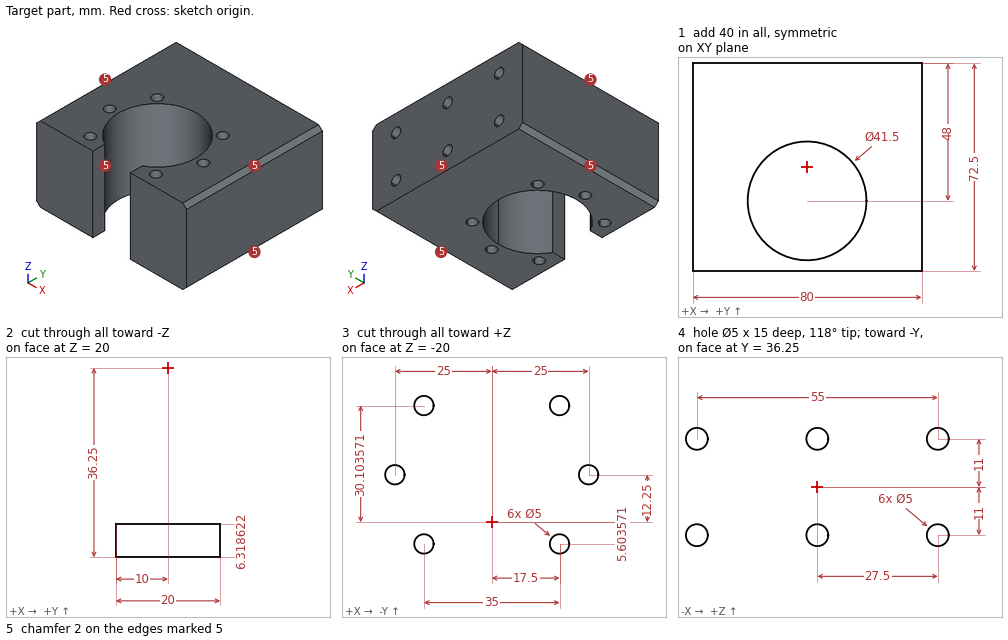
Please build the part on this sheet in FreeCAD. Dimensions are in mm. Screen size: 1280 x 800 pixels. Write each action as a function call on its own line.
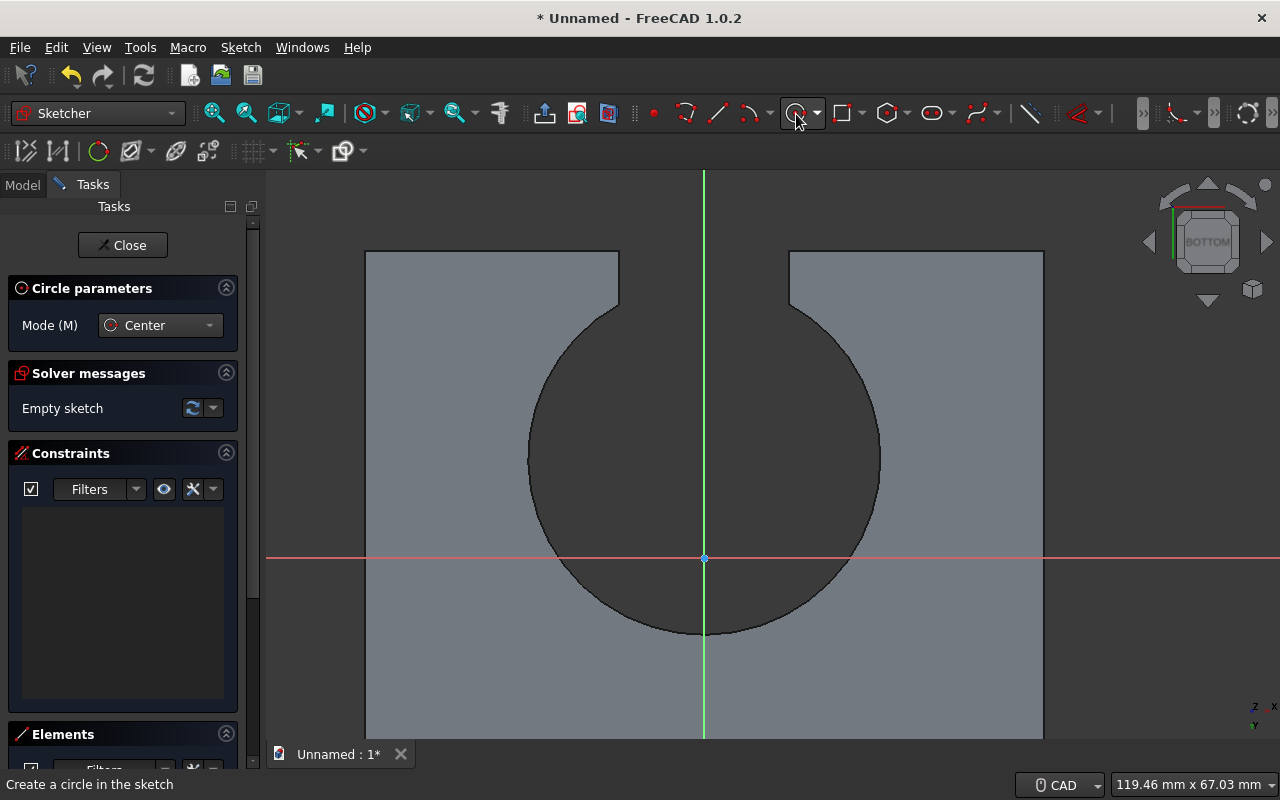
click(853, 606)
move(868, 591)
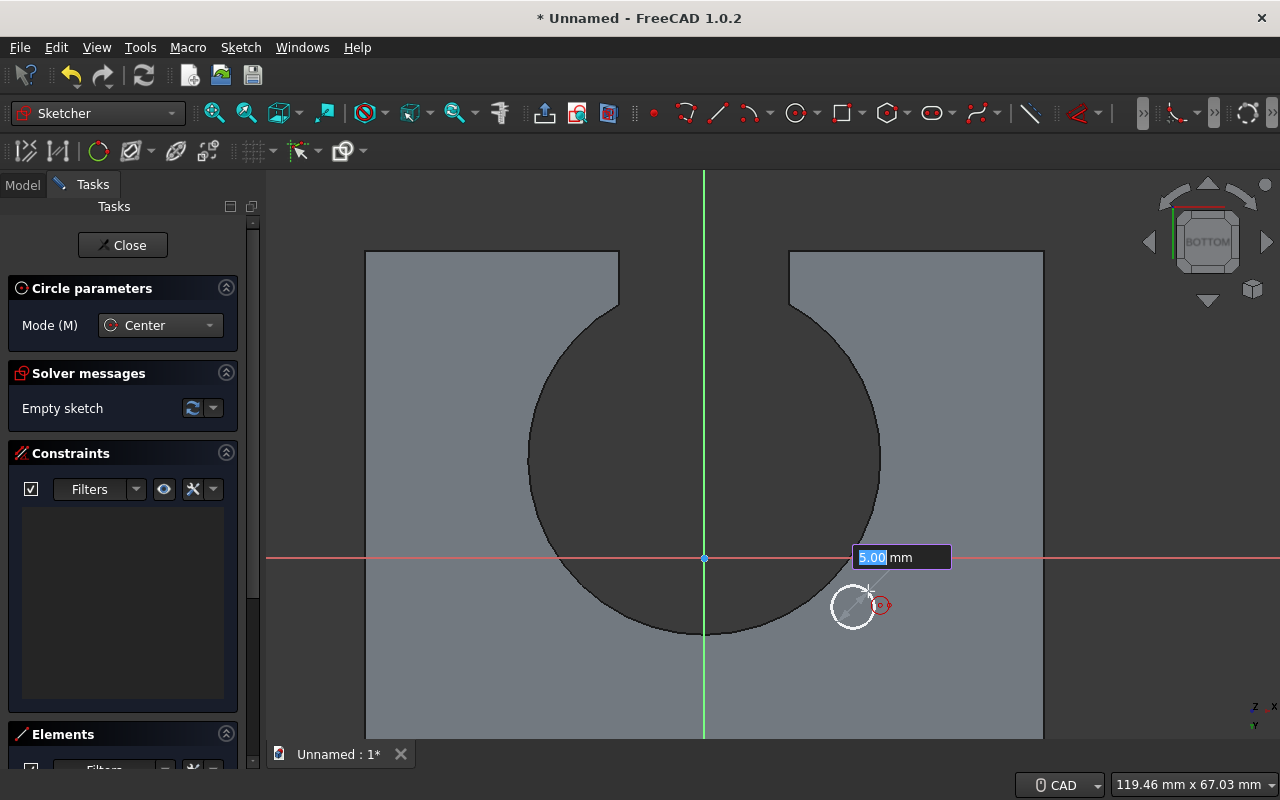
text(5)
key(Return)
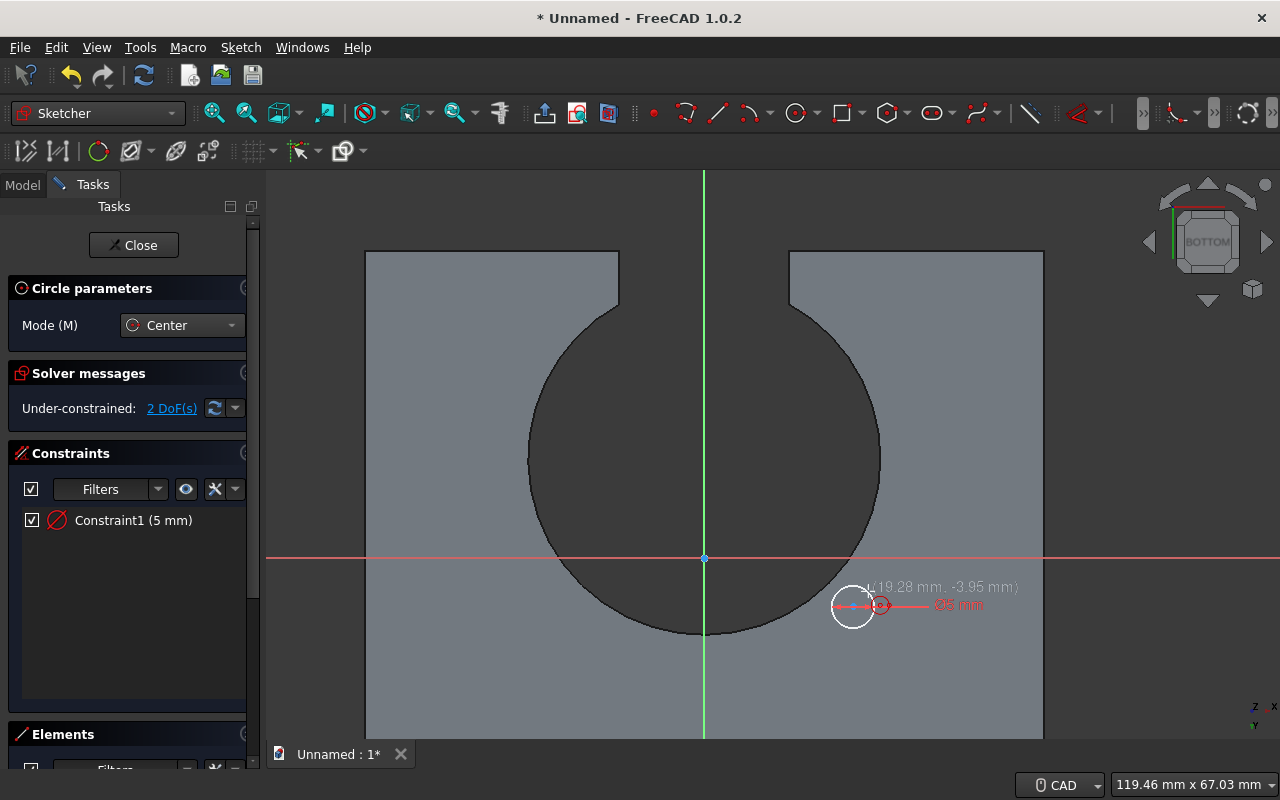
click(556, 606)
move(571, 591)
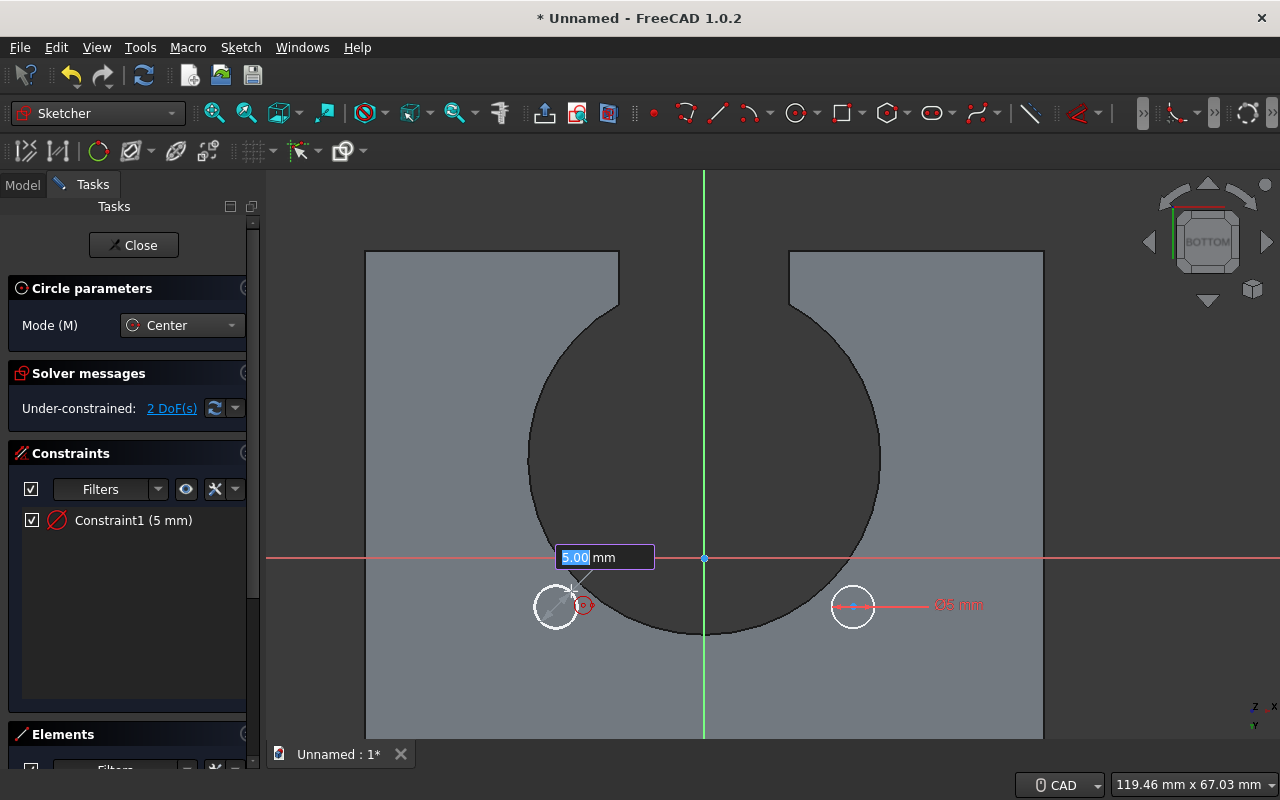
text(5)
key(Return)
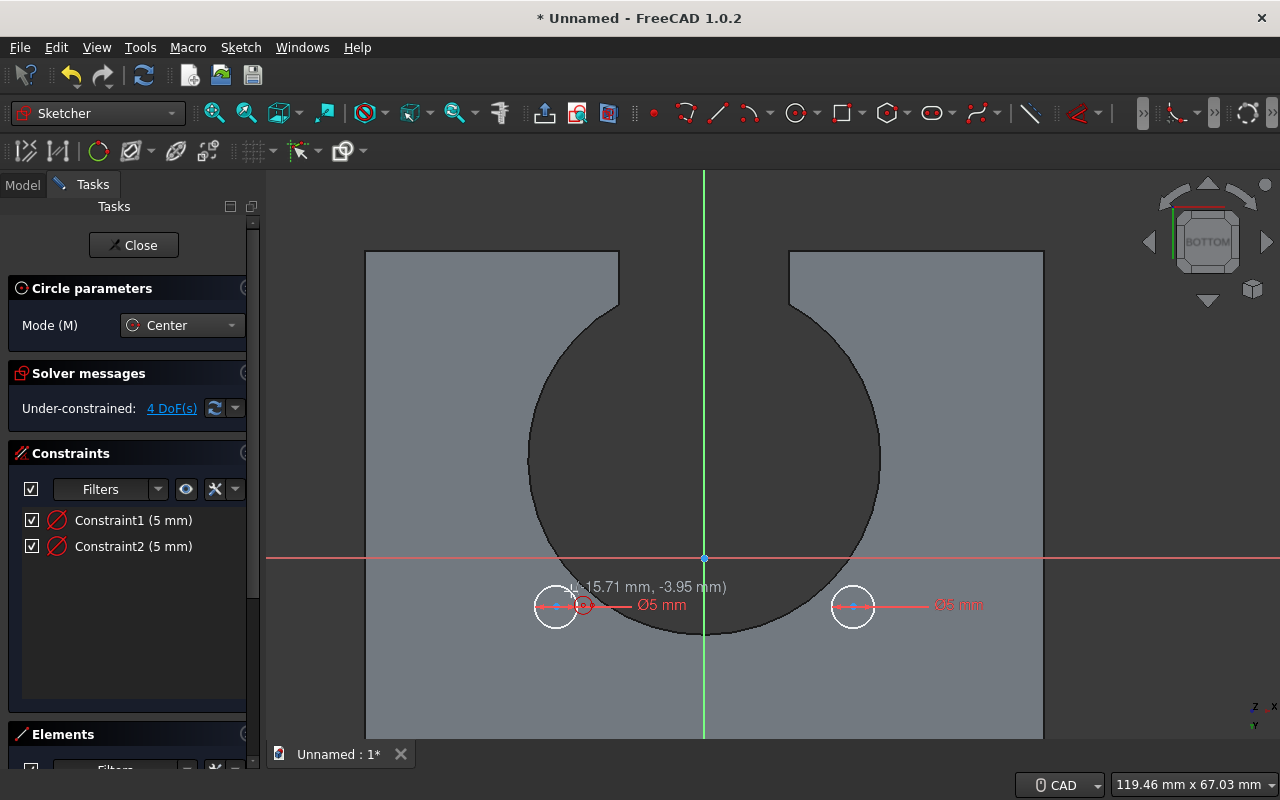
click(556, 303)
move(571, 288)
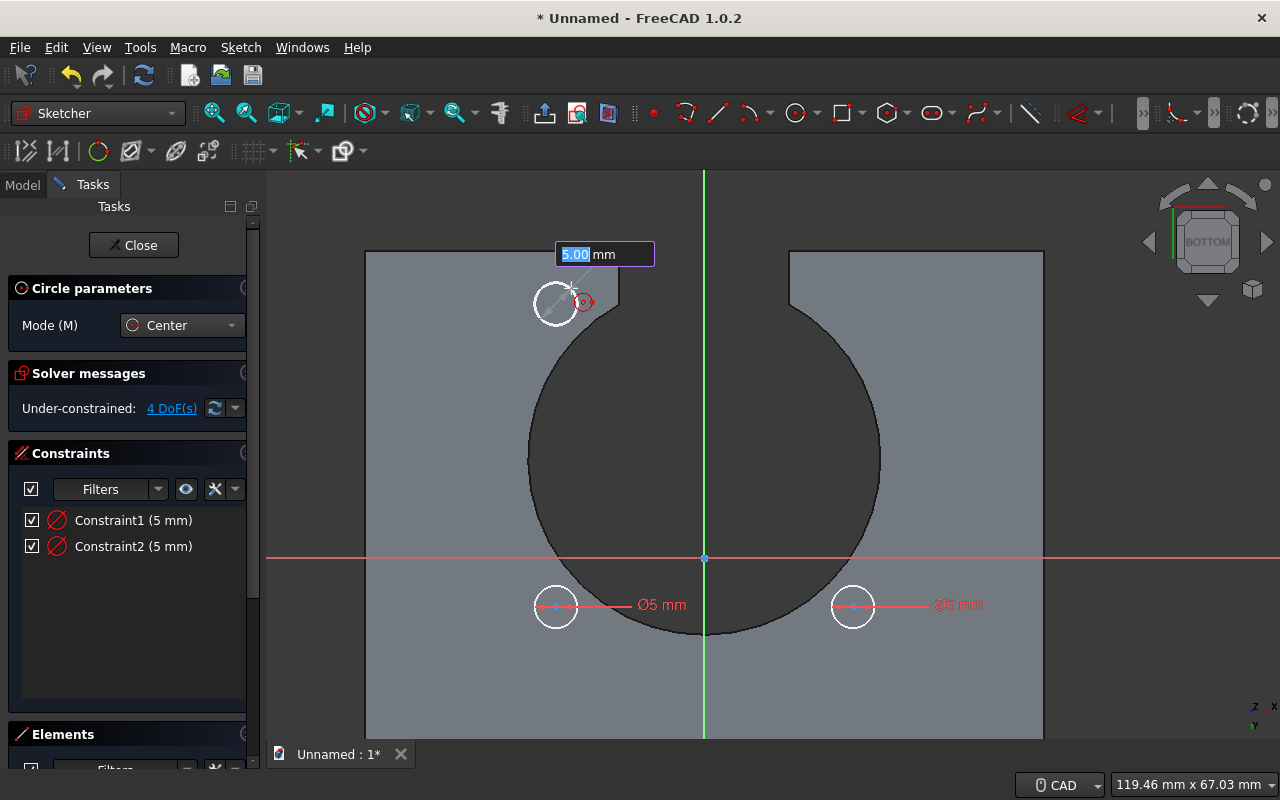
text(5)
key(Return)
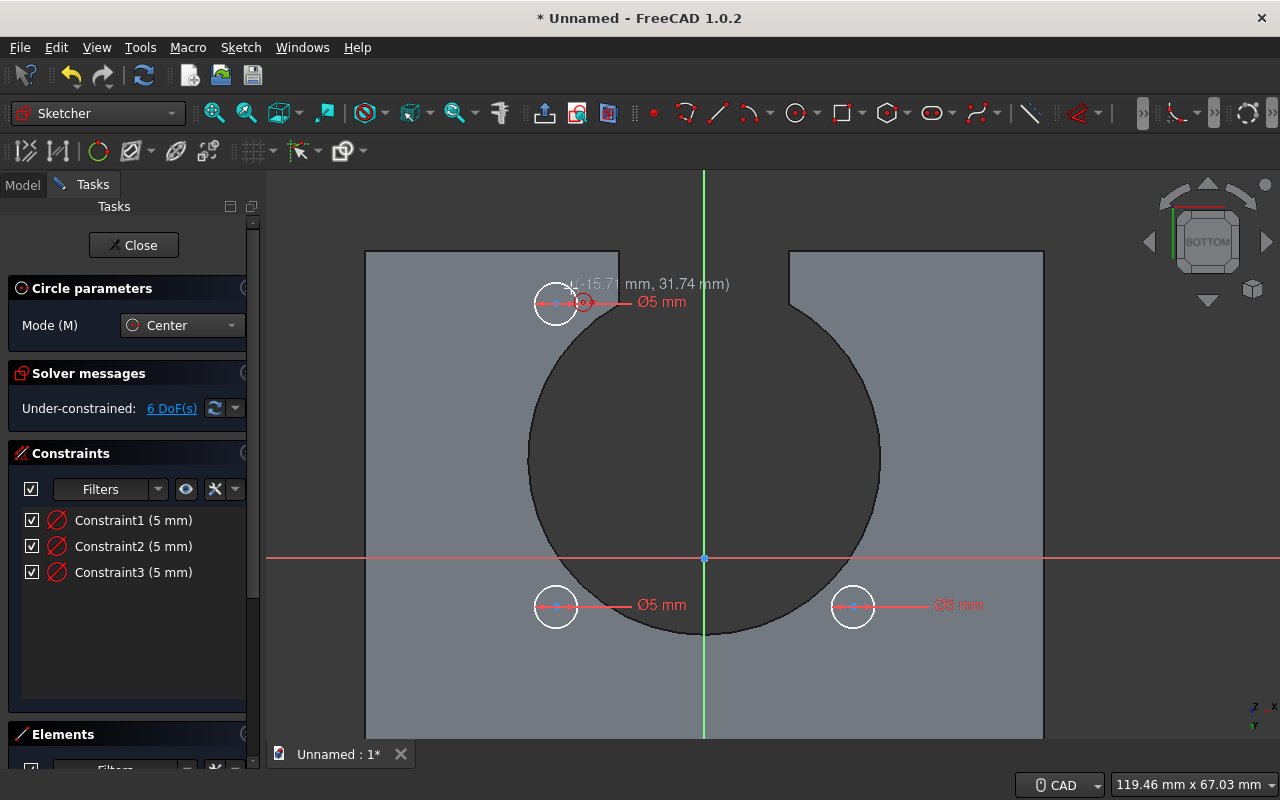
click(853, 303)
move(868, 288)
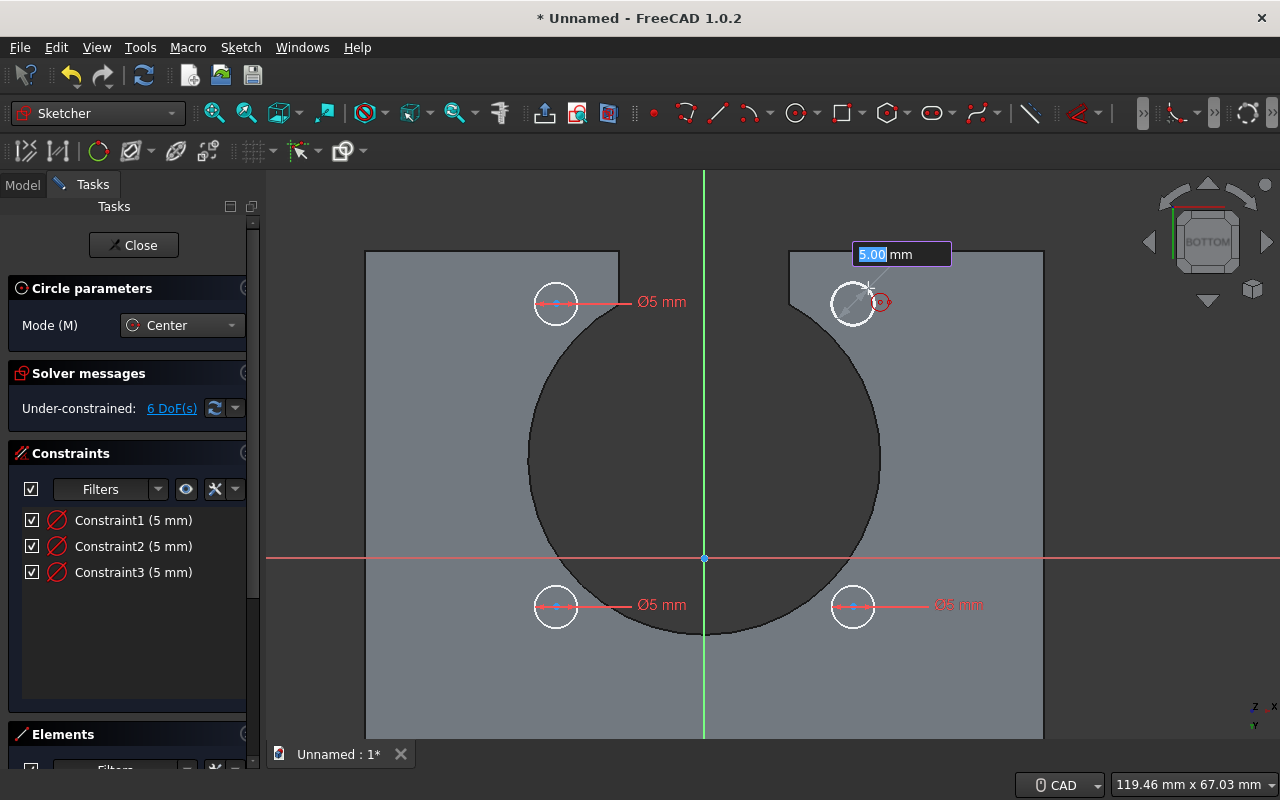
text(5)
key(Return)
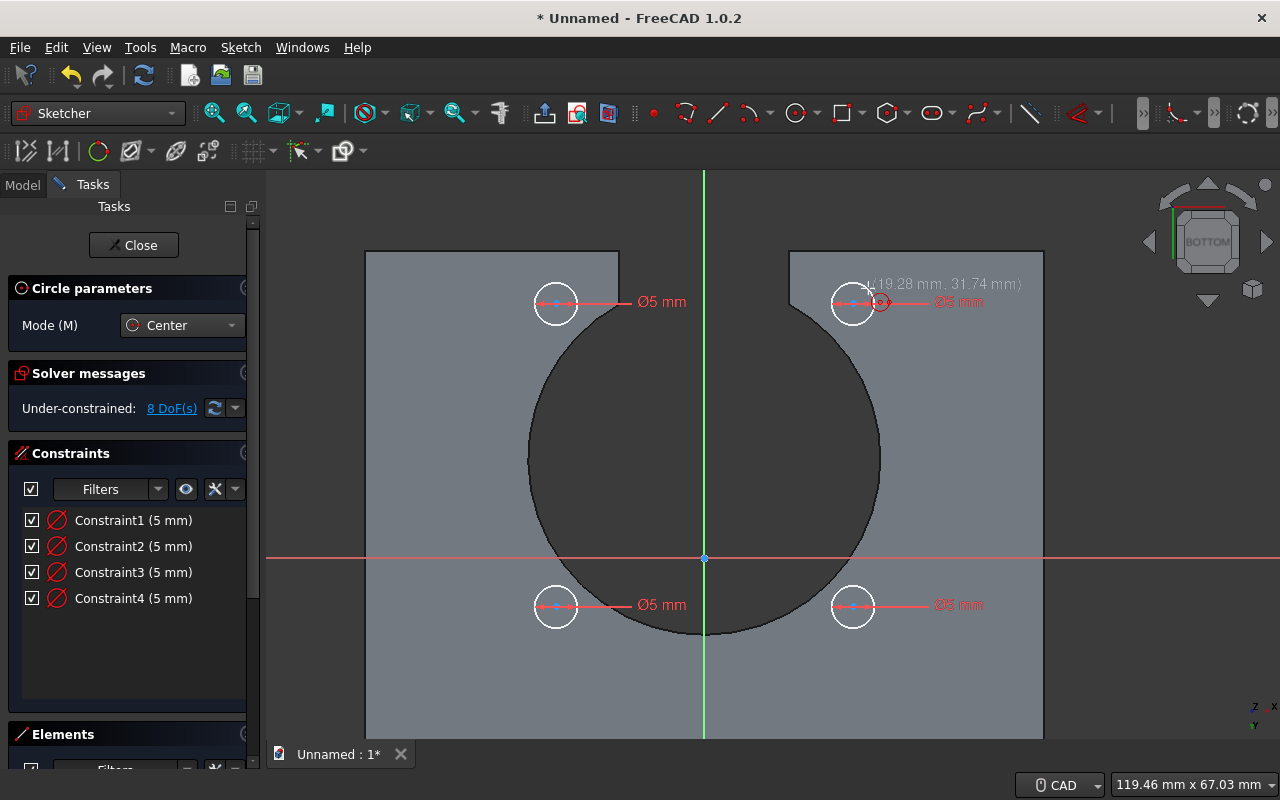
click(917, 454)
move(932, 439)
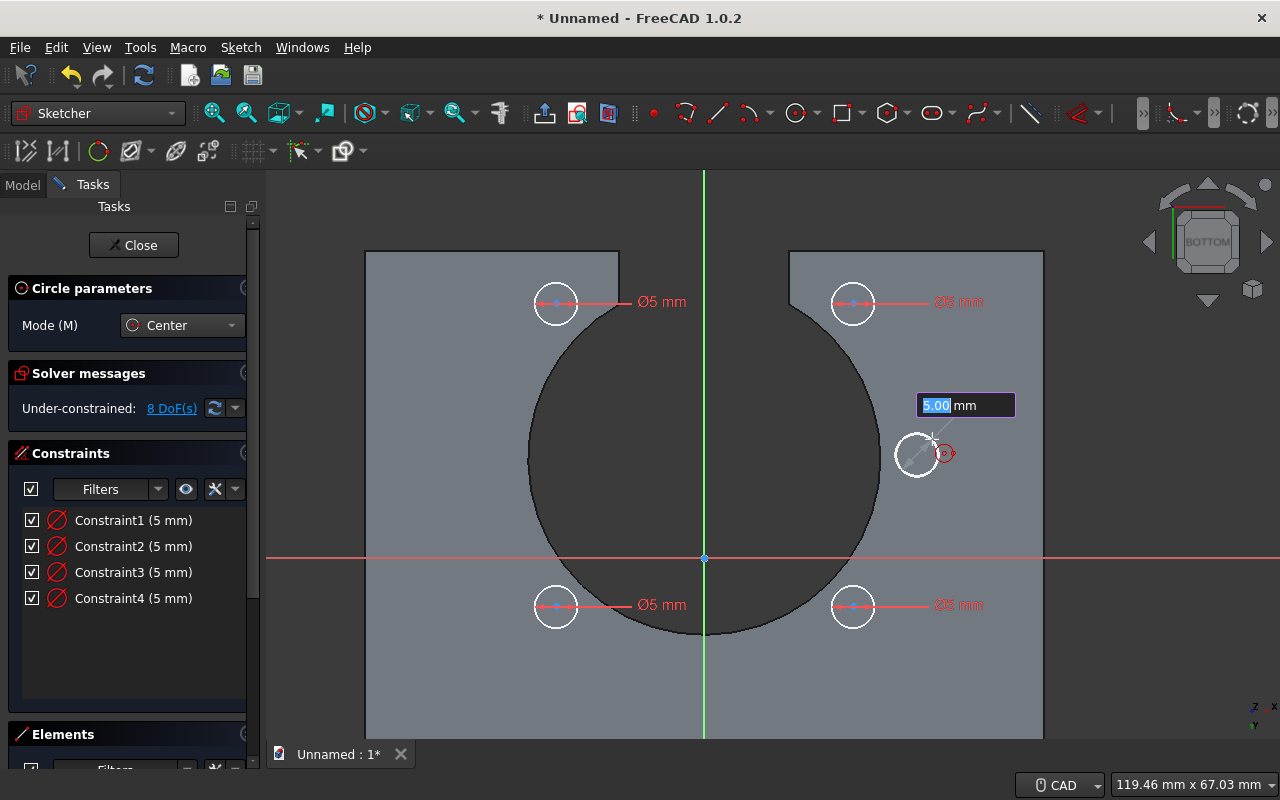
text(5)
key(Return)